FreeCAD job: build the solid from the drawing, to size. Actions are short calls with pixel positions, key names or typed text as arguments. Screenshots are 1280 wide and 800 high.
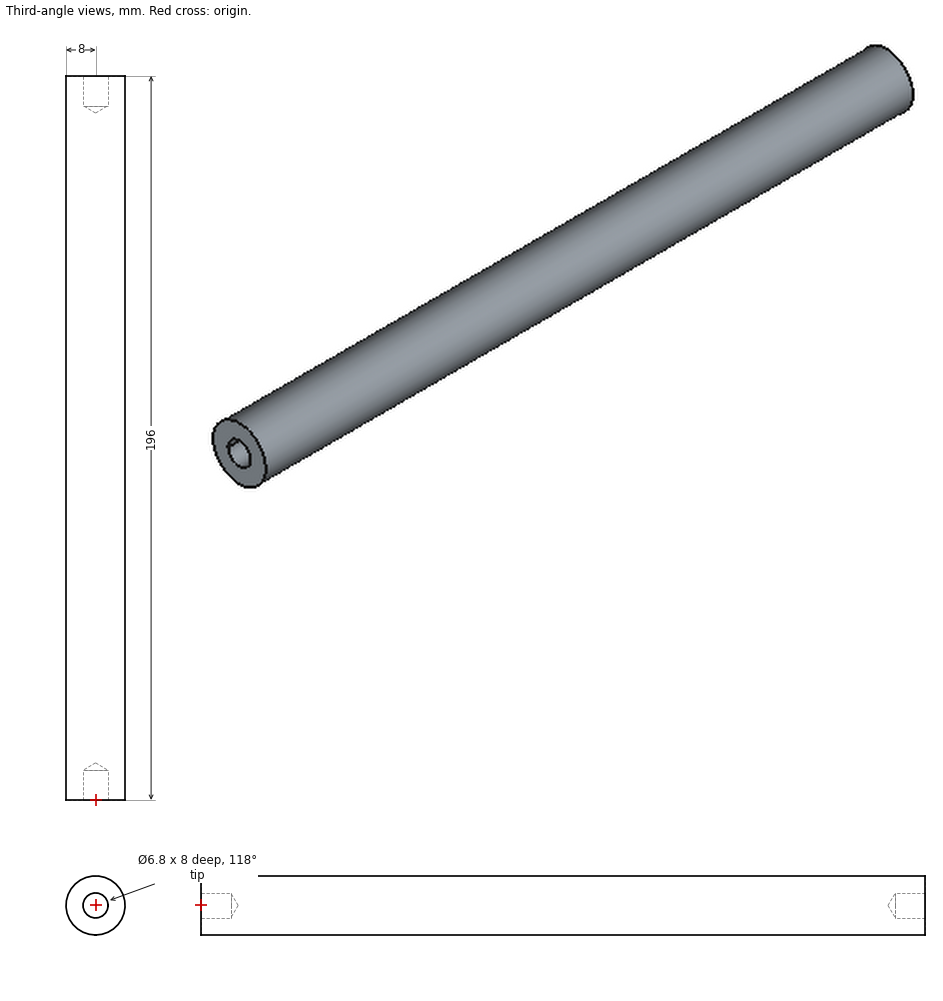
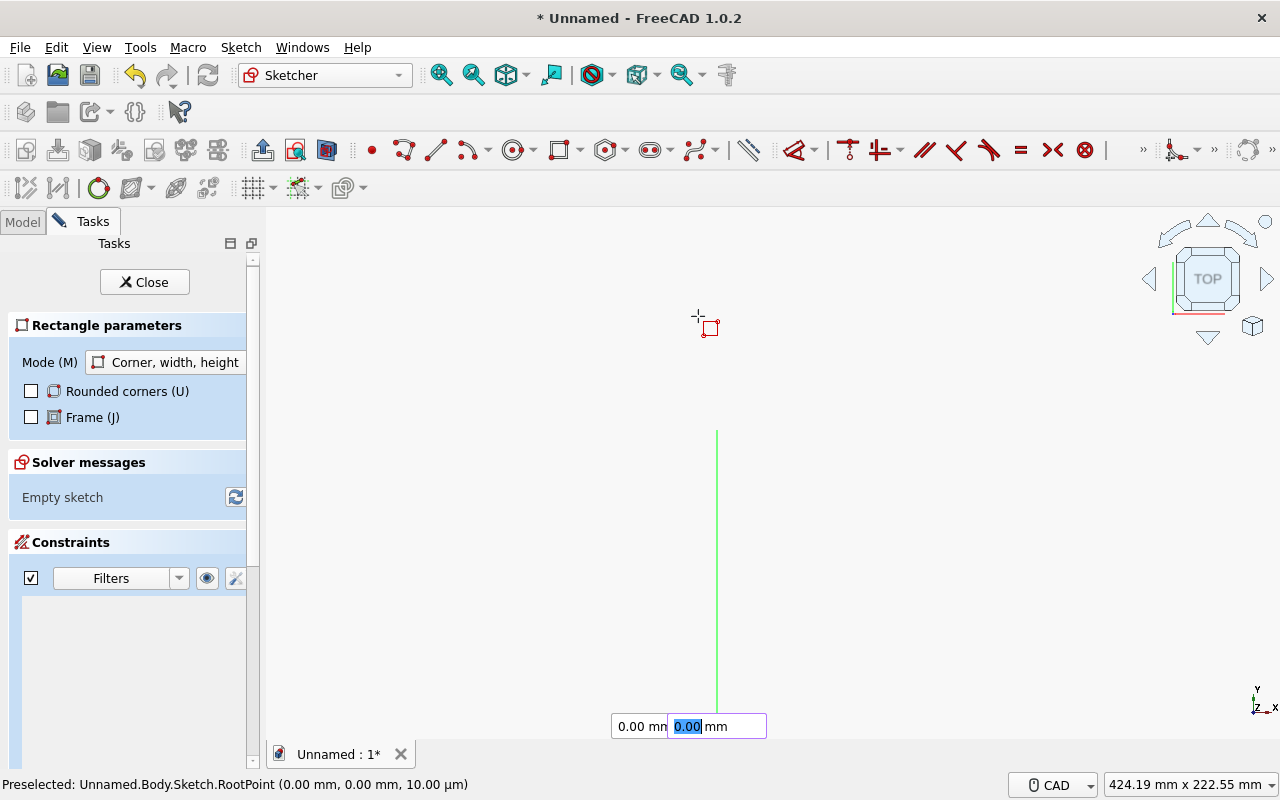
click(698, 316)
key(Escape)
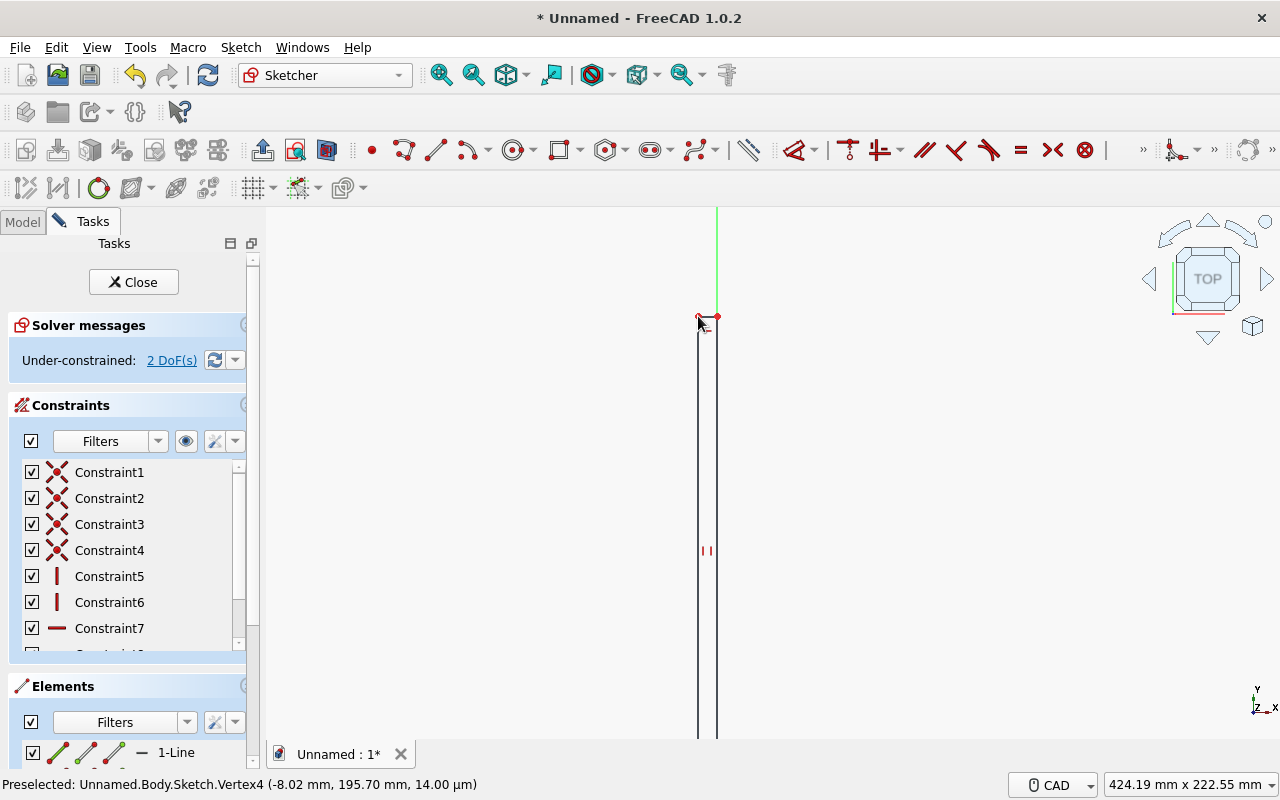
click(794, 150)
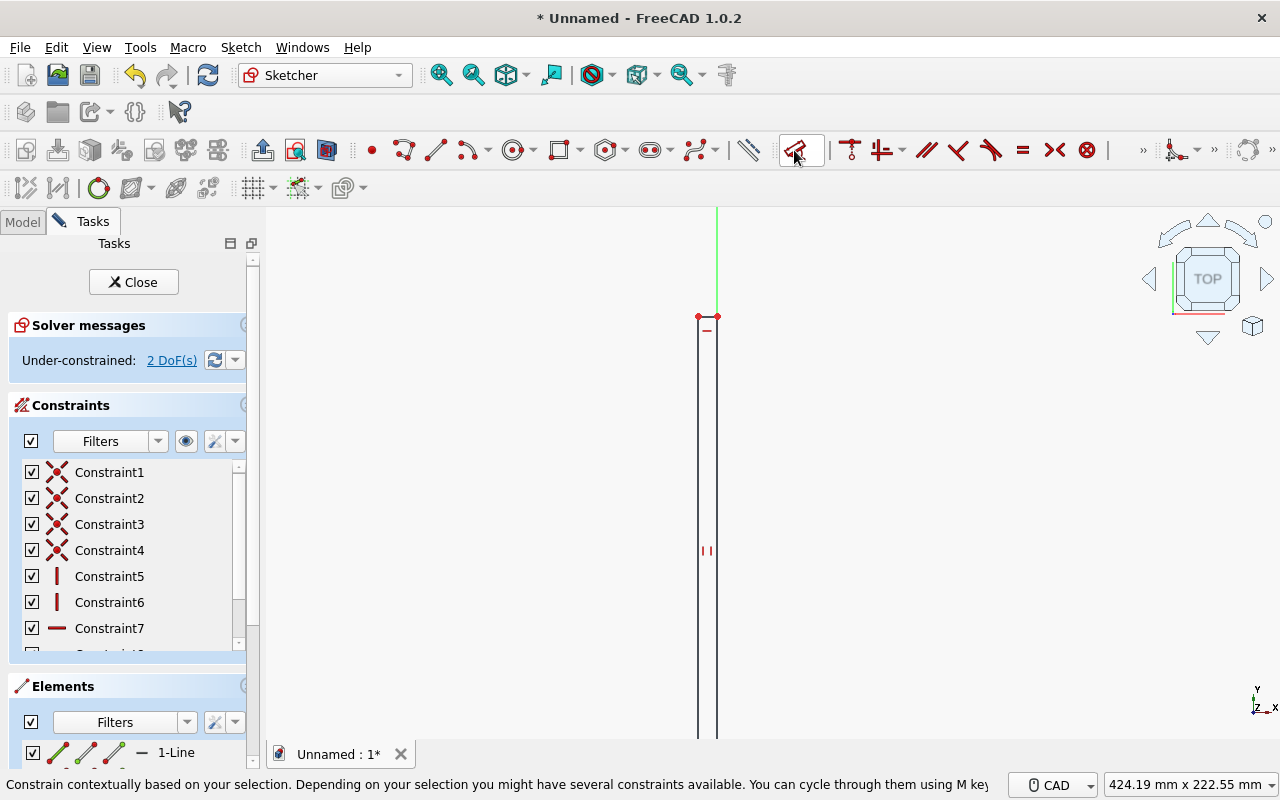
scroll(708, 317, up, 4)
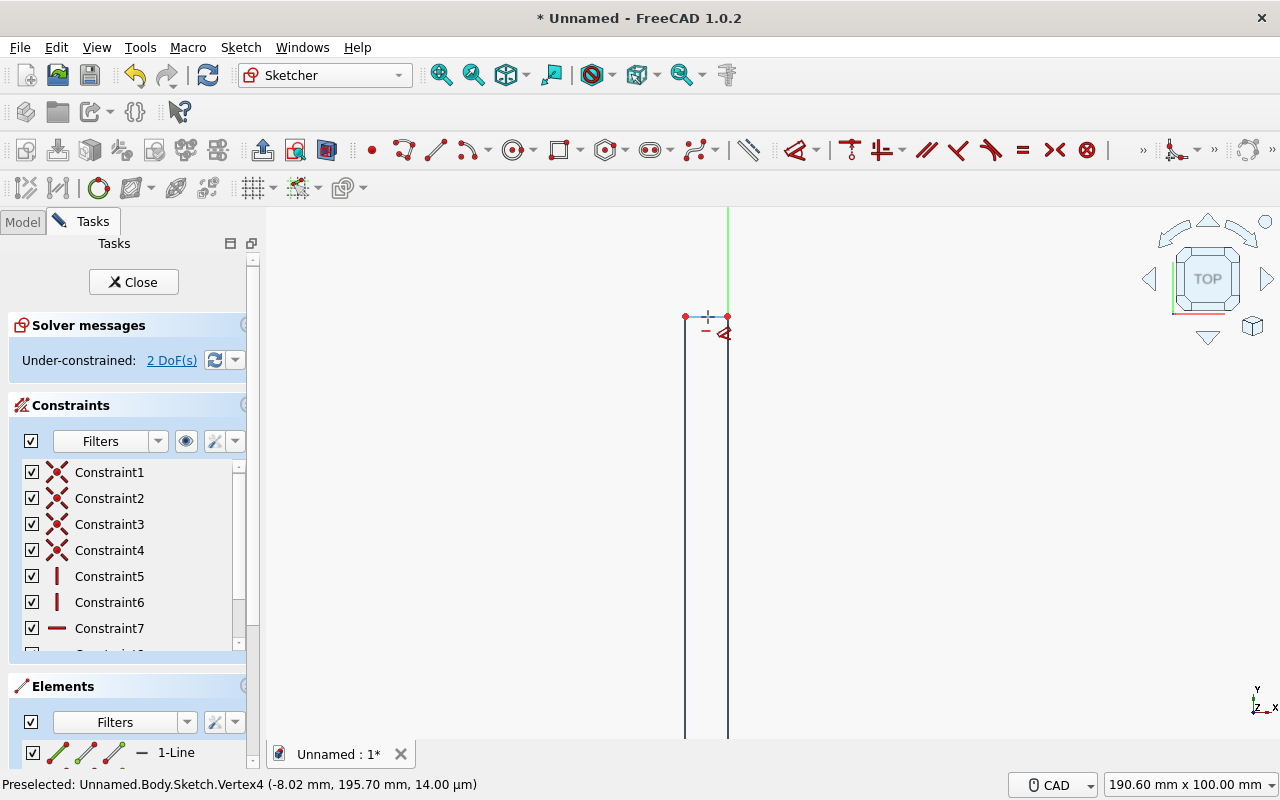
click(707, 317)
click(707, 283)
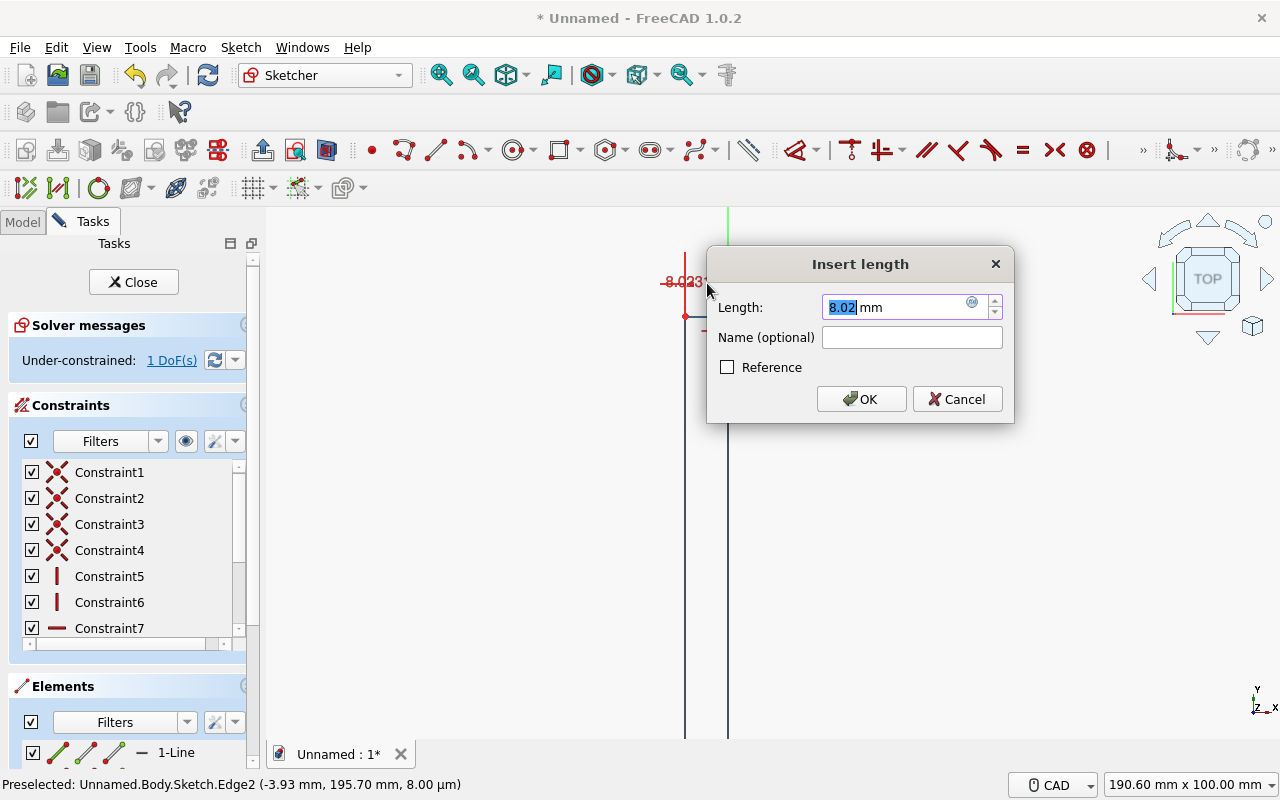
text(8)
key(Return)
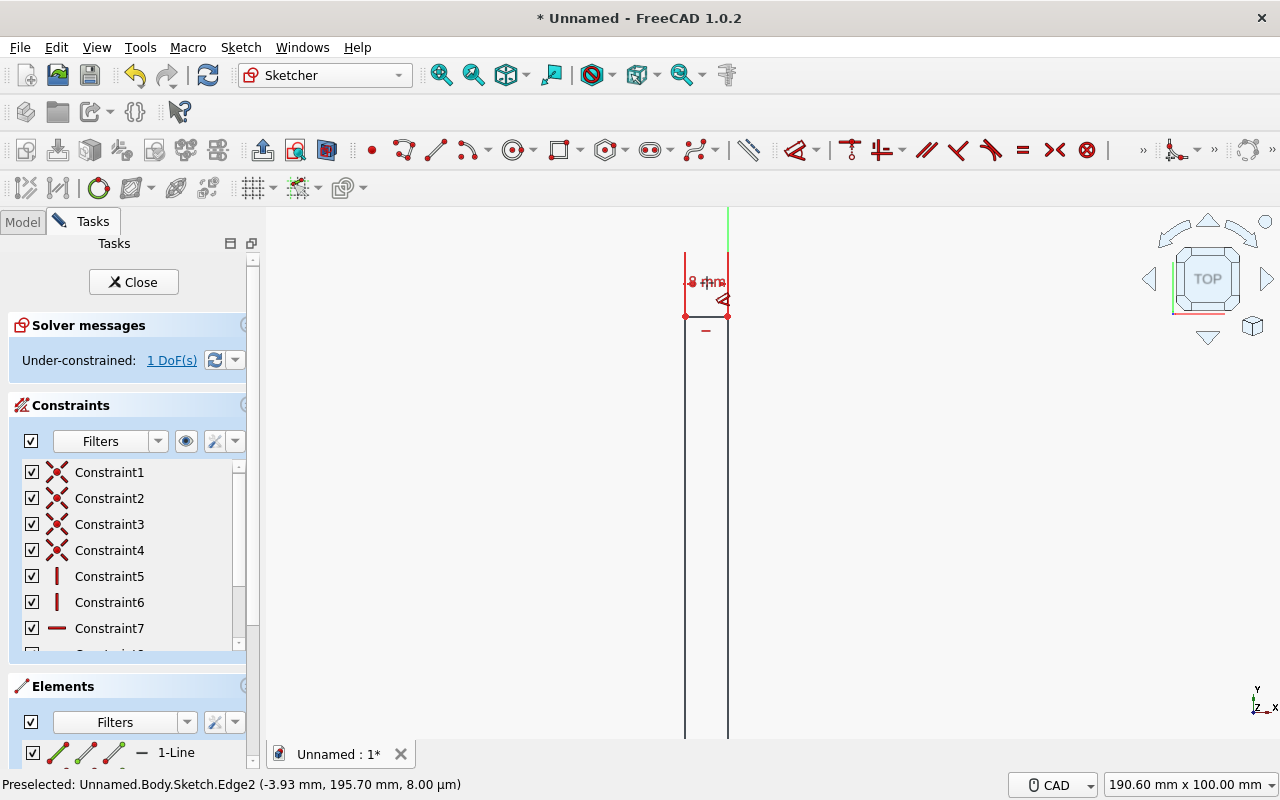
click(728, 629)
click(762, 514)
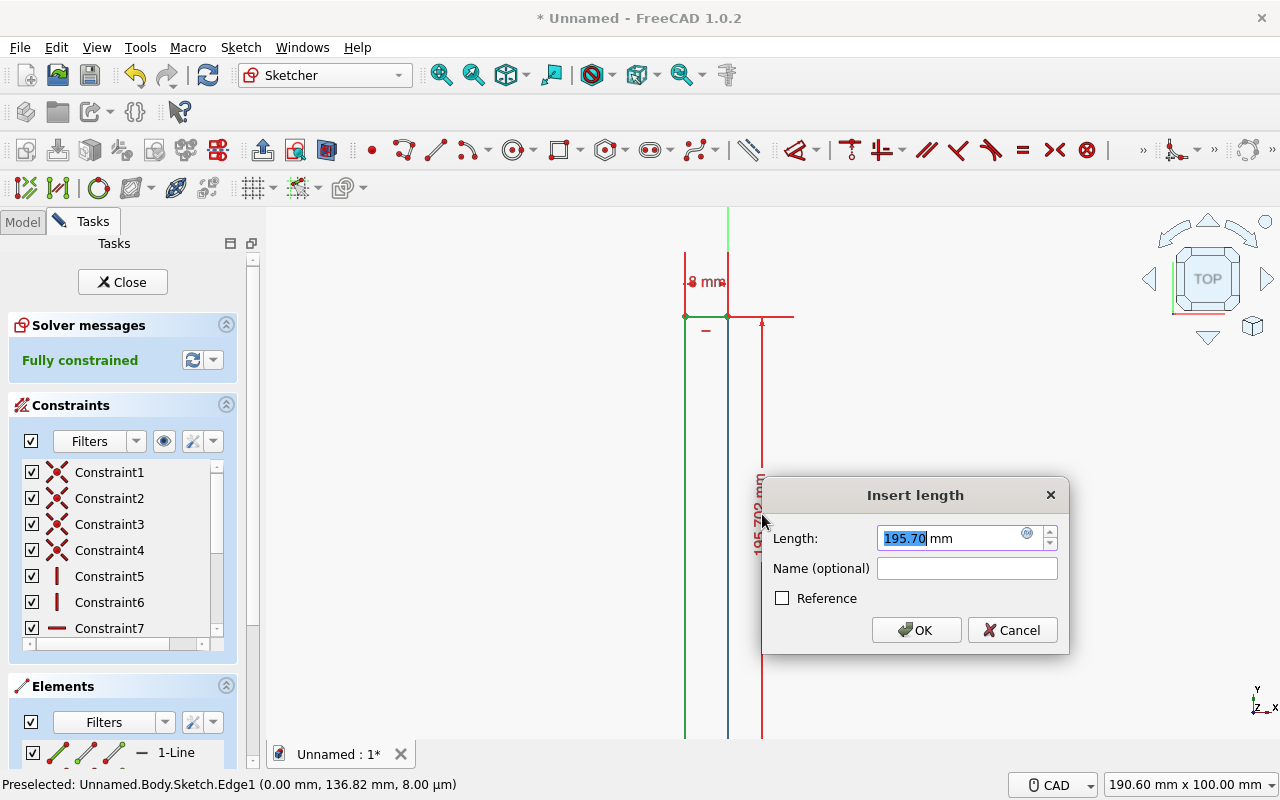
text(196)
key(Return)
key(Escape)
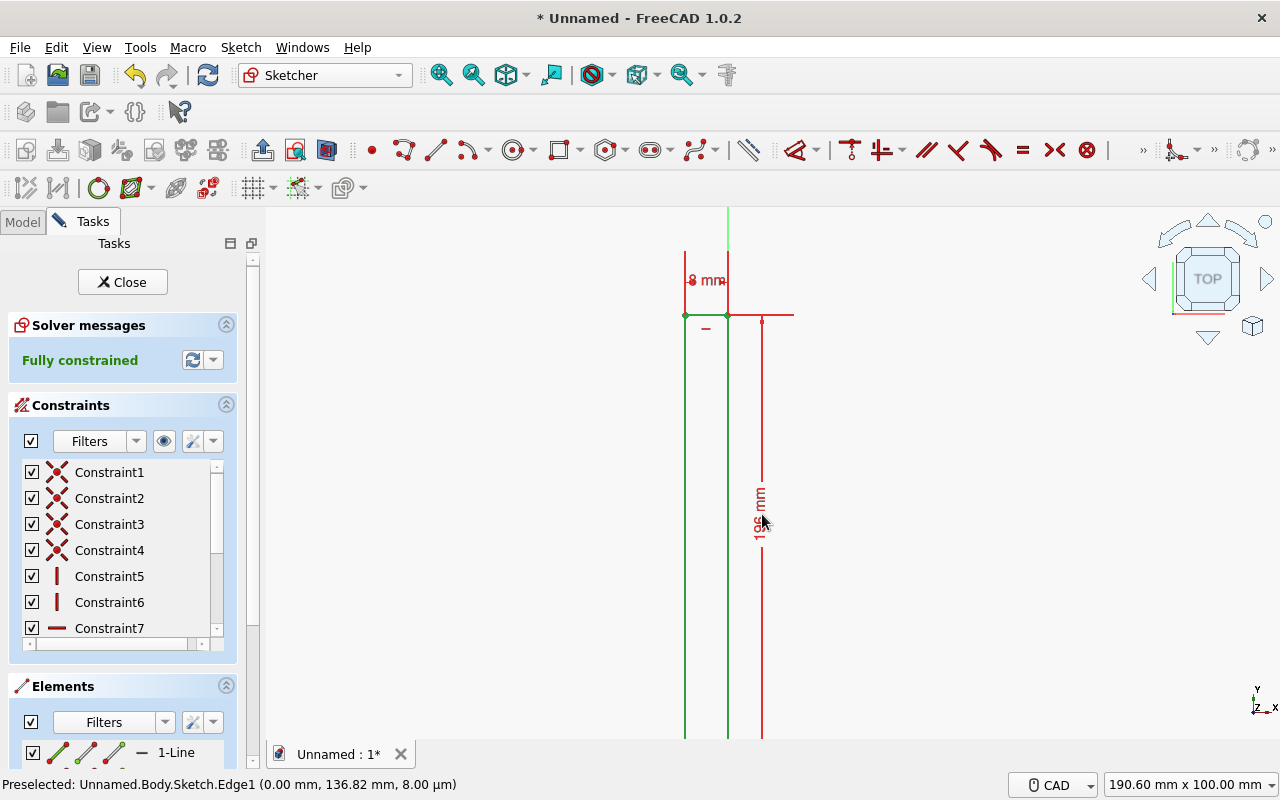
click(123, 282)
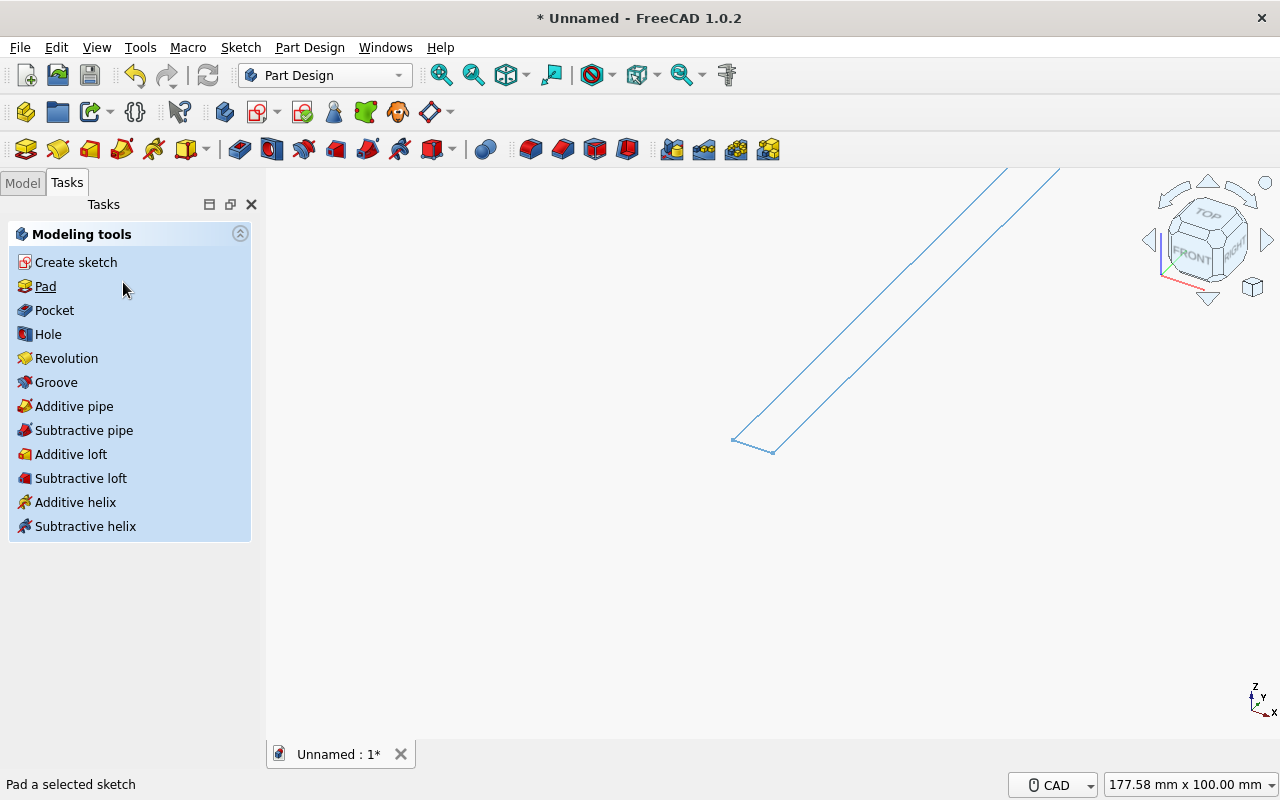
click(58, 150)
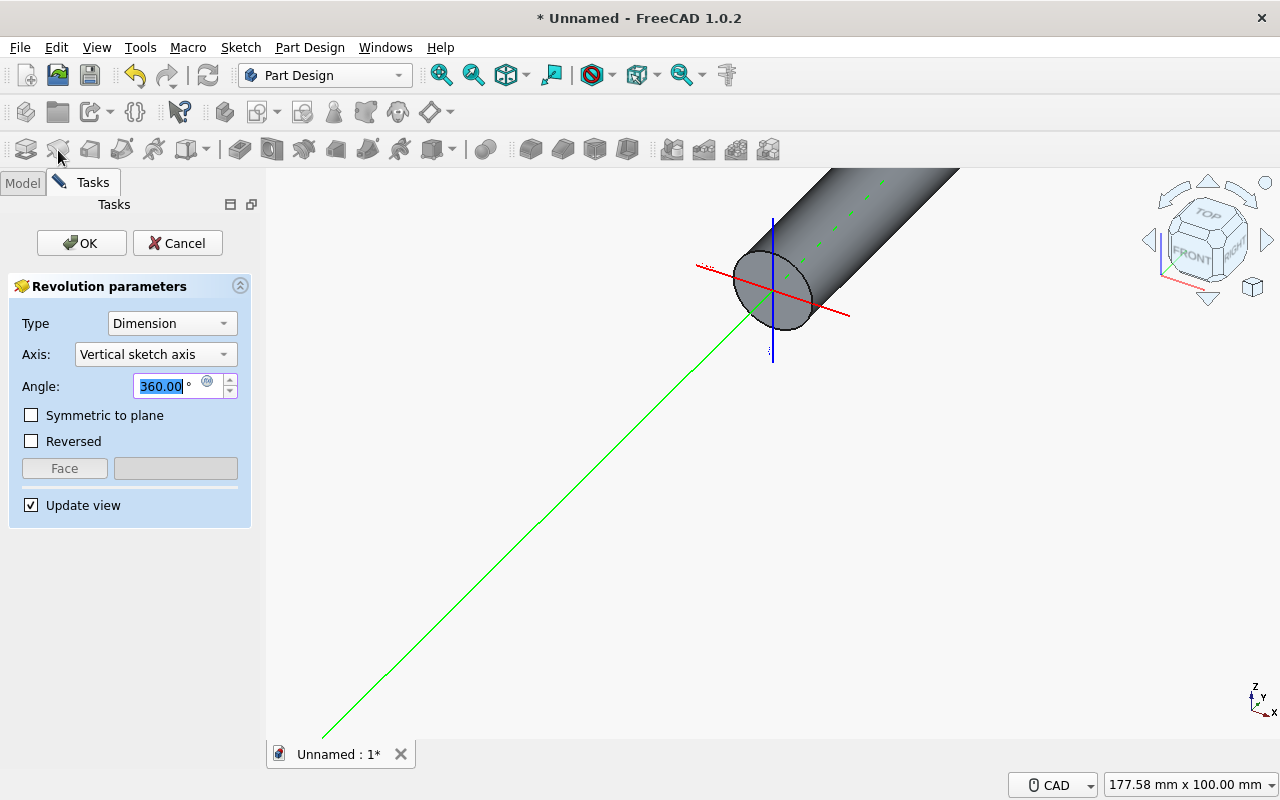
click(82, 243)